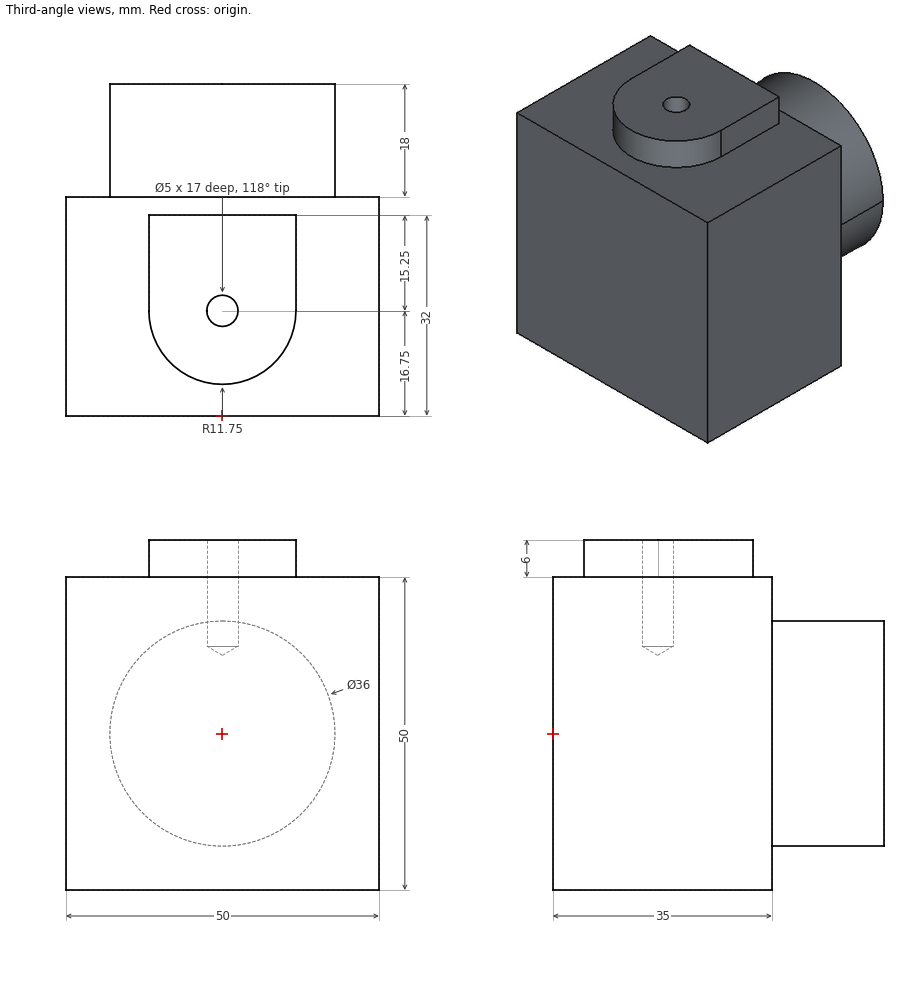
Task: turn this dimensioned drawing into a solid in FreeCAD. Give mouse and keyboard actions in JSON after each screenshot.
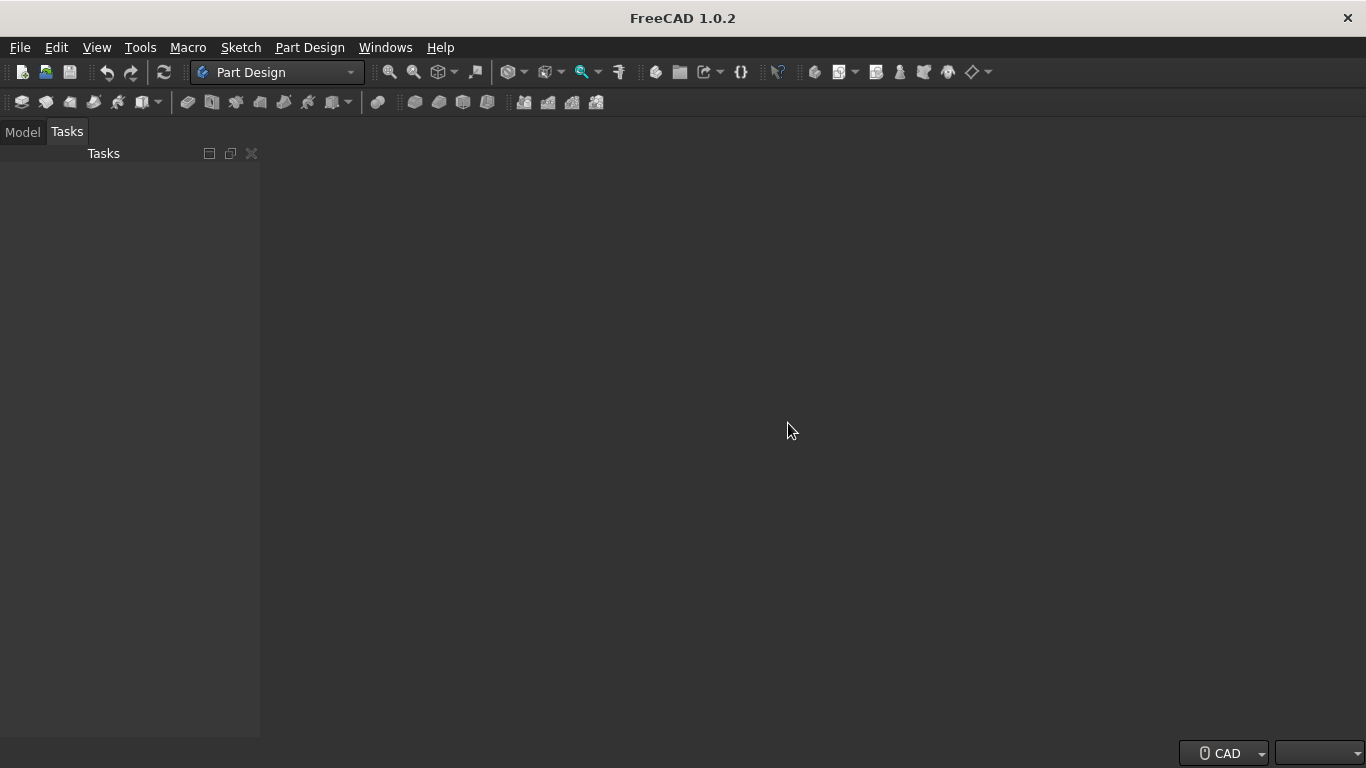
{"action": "key", "text": "ctrl+n"}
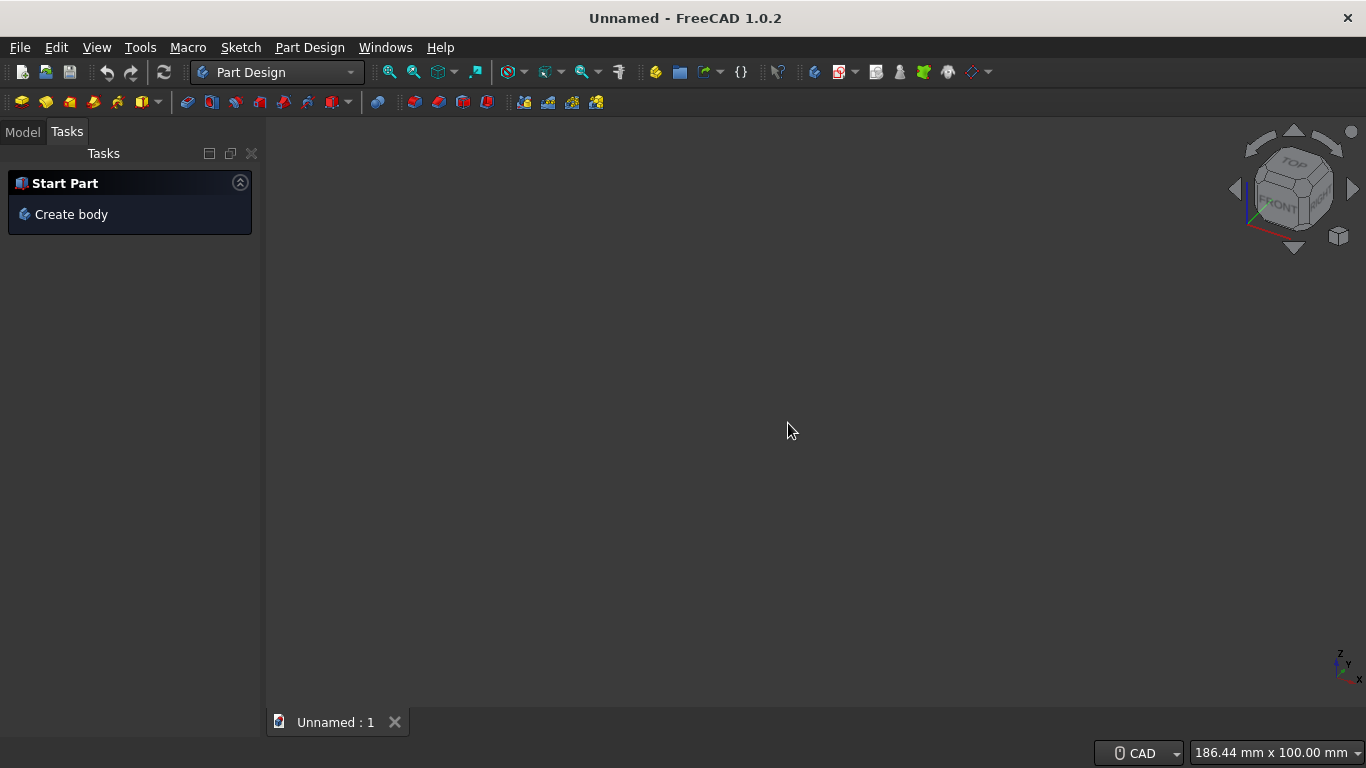
{"action": "left_click", "coordinate": [840, 72]}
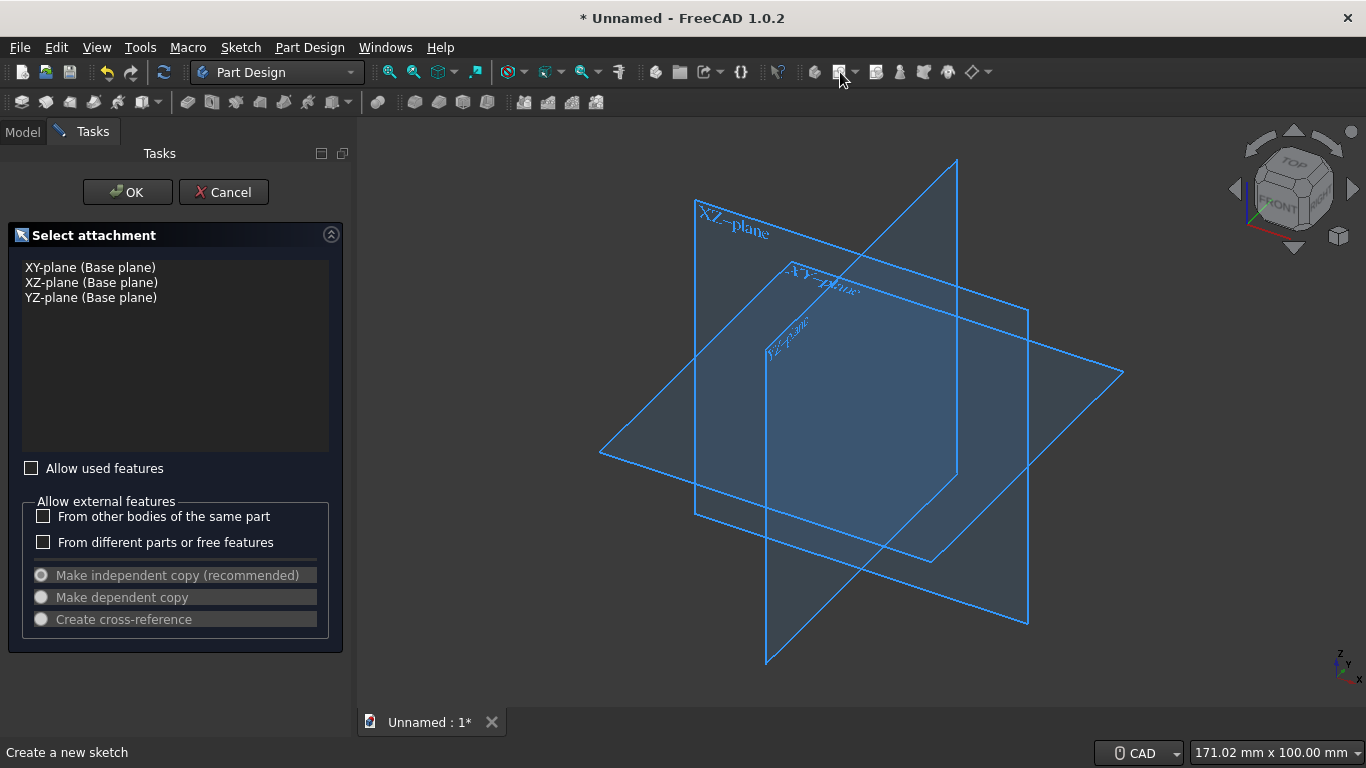
{"action": "left_click", "coordinate": [82, 282]}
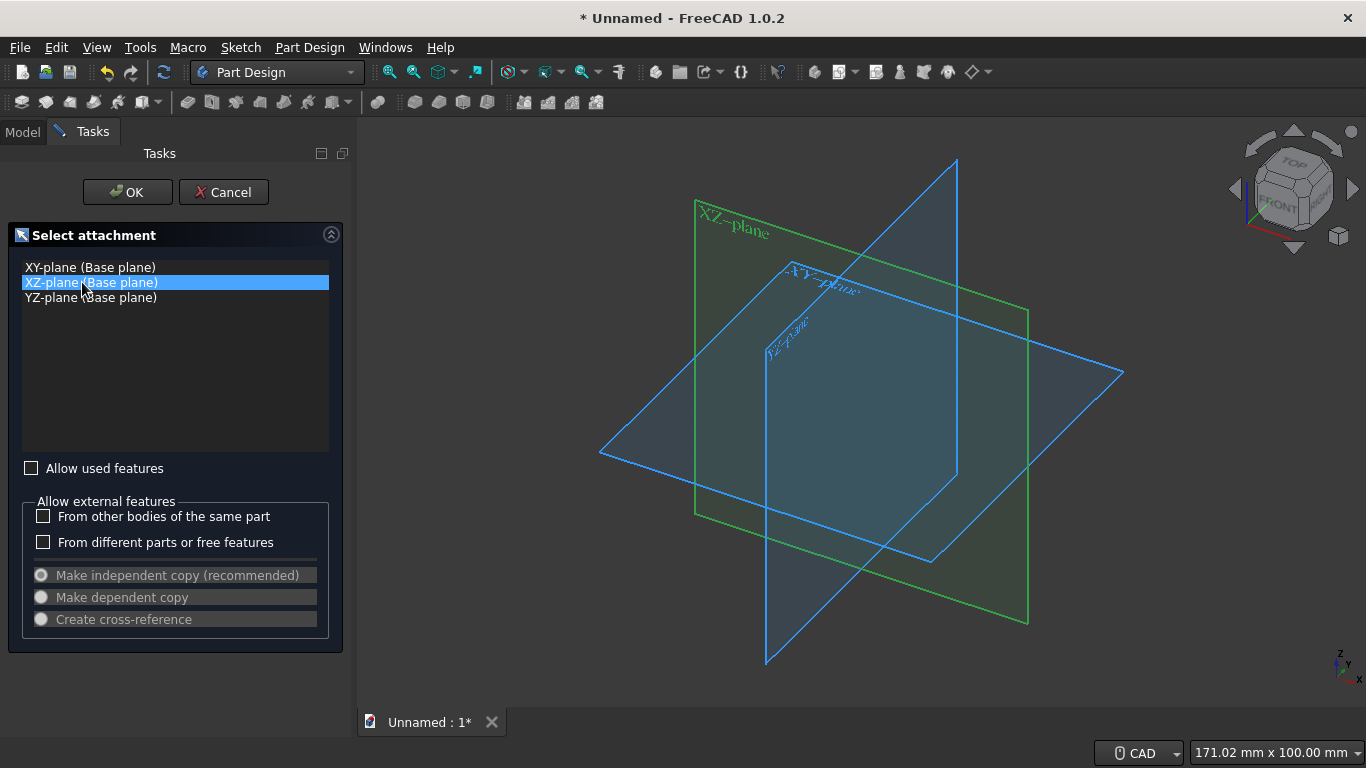
{"action": "left_click", "coordinate": [128, 192]}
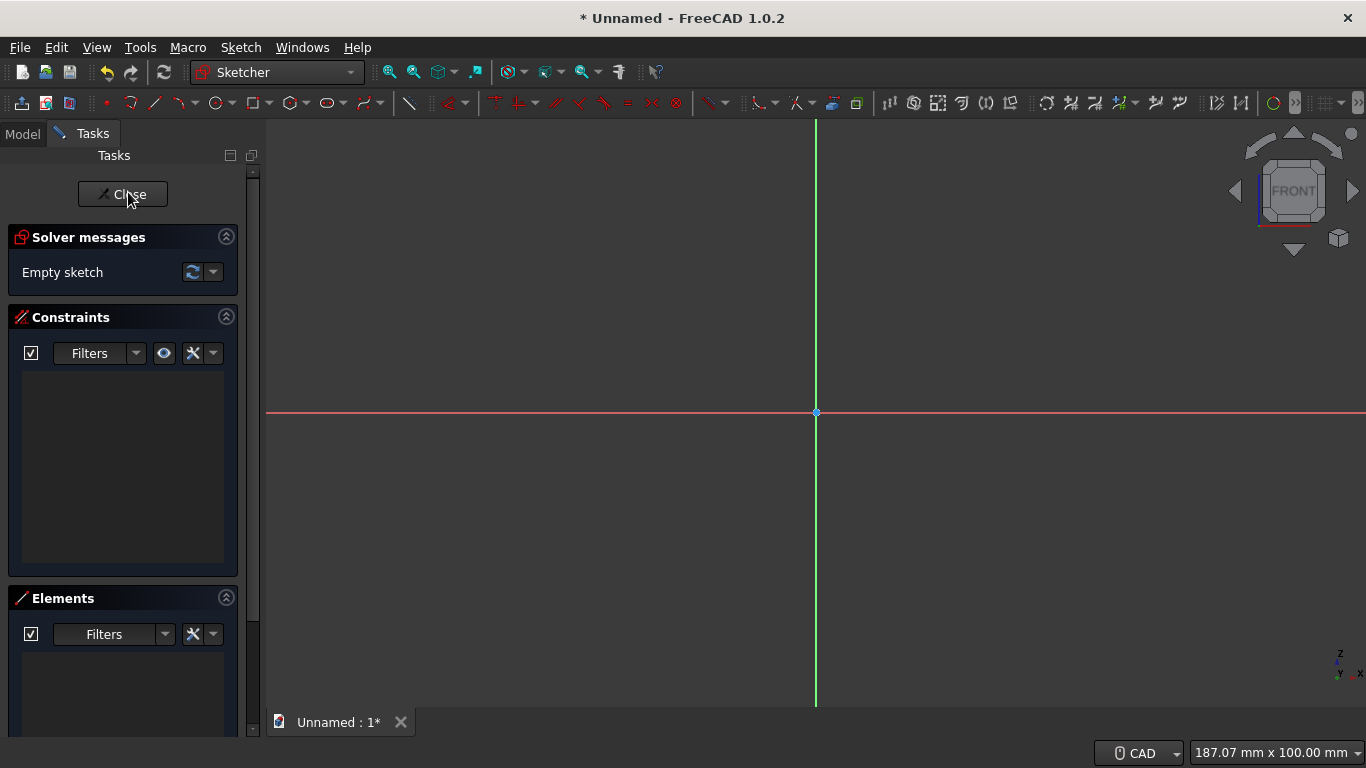
{"action": "key", "text": "g v"}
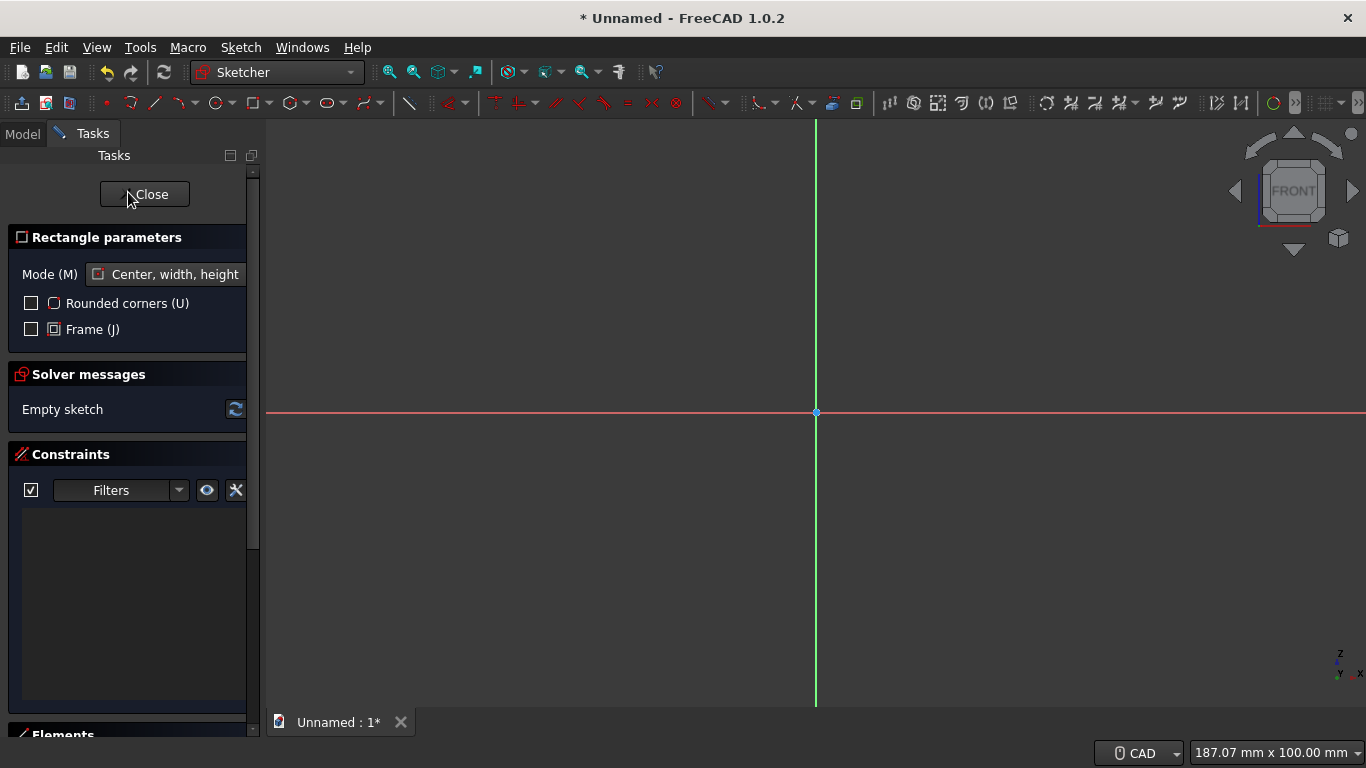
{"action": "left_click", "coordinate": [816, 413]}
{"action": "left_click", "coordinate": [963, 266]}
{"action": "key", "text": "Escape"}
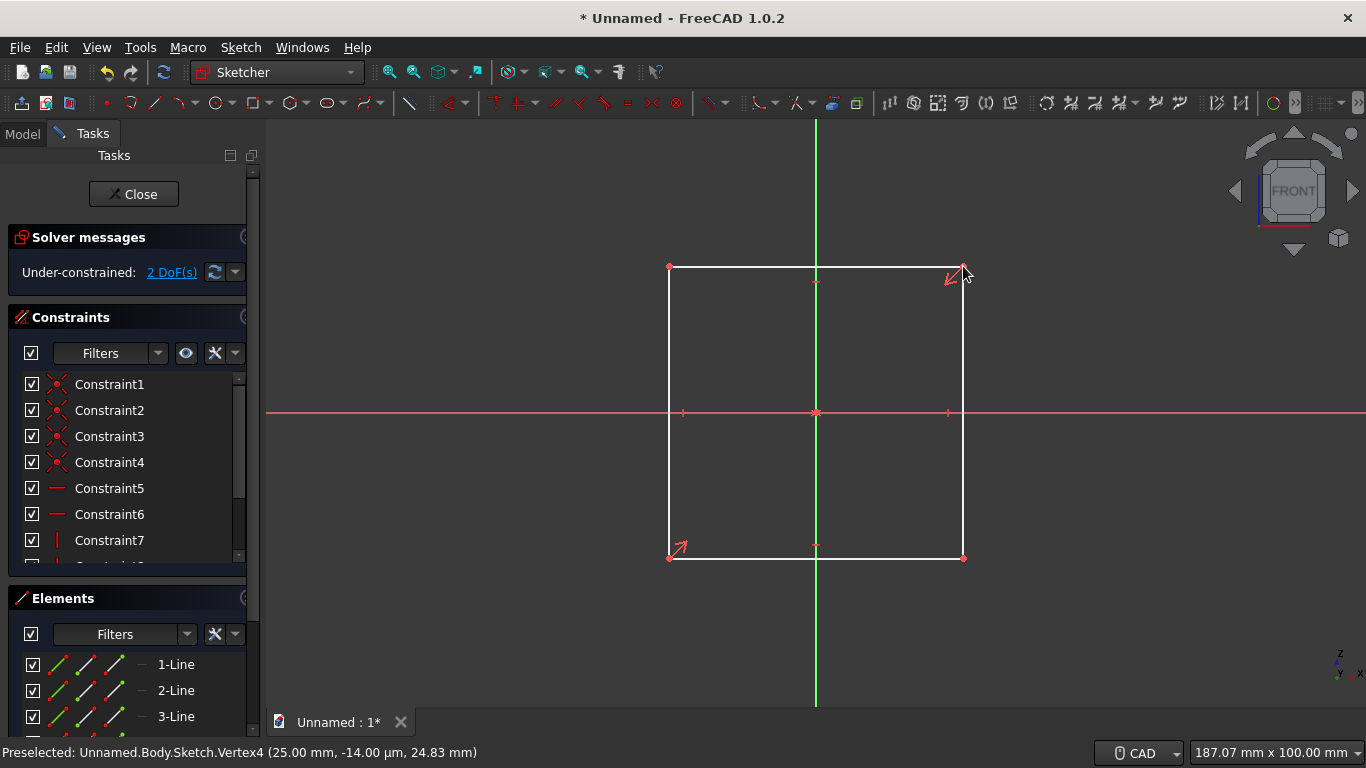
{"action": "left_click", "coordinate": [448, 104]}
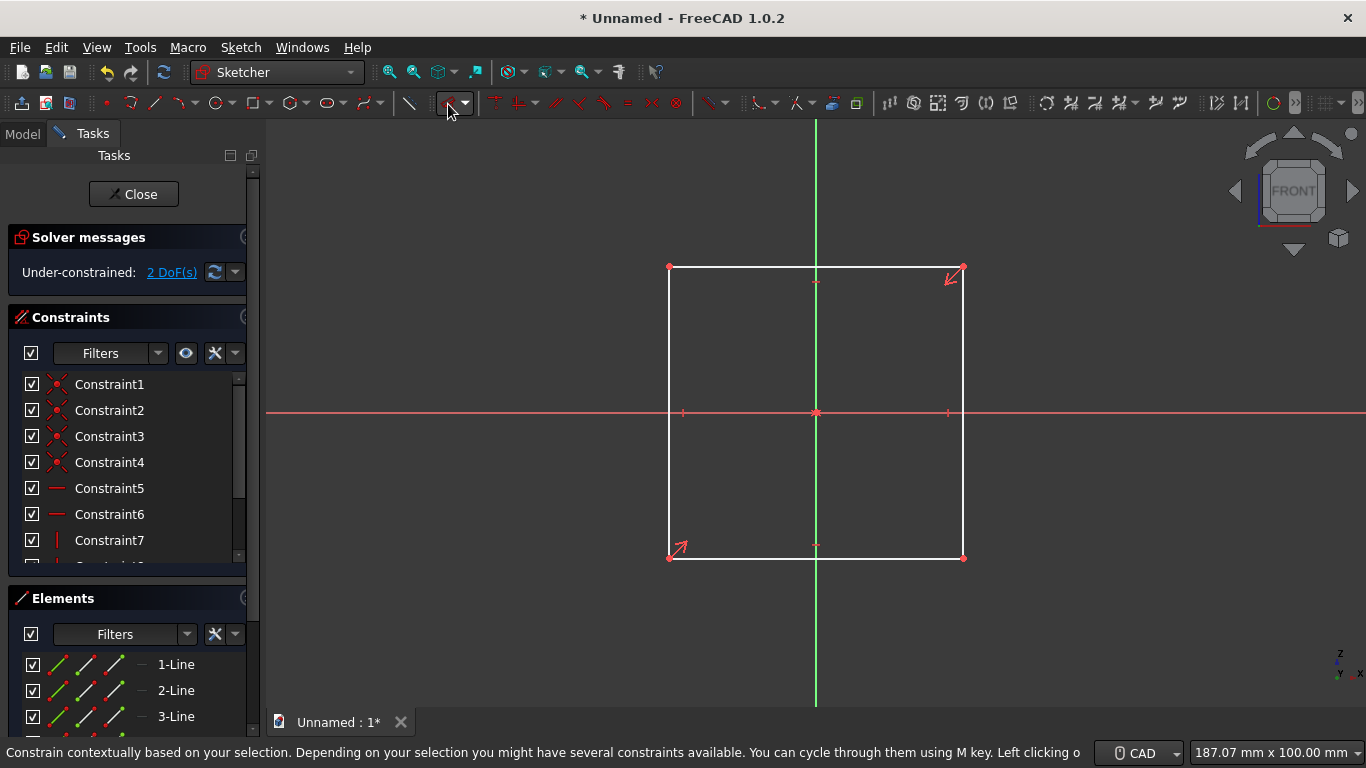
{"action": "left_click", "coordinate": [757, 559]}
{"action": "left_click", "coordinate": [748, 593]}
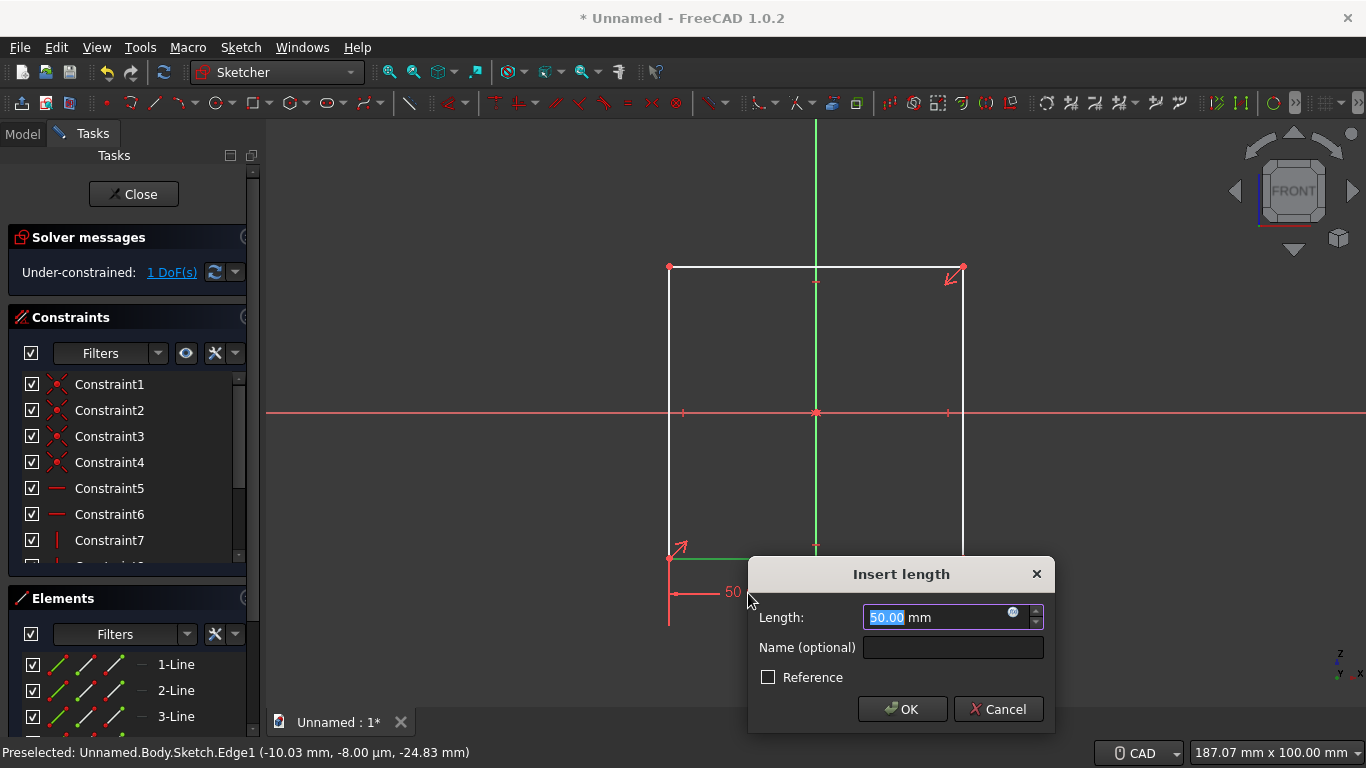
{"action": "type", "text": "50"}
{"action": "key", "text": "Return"}